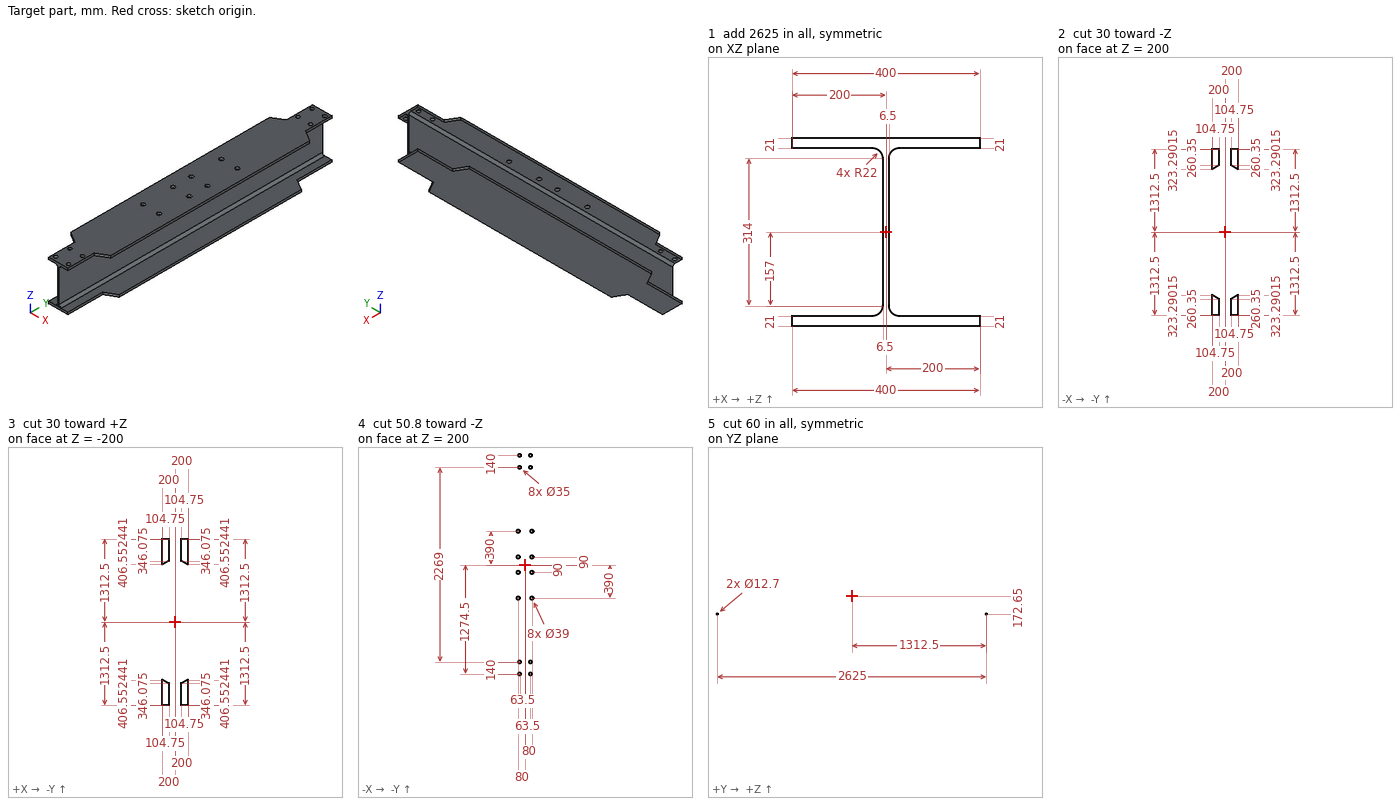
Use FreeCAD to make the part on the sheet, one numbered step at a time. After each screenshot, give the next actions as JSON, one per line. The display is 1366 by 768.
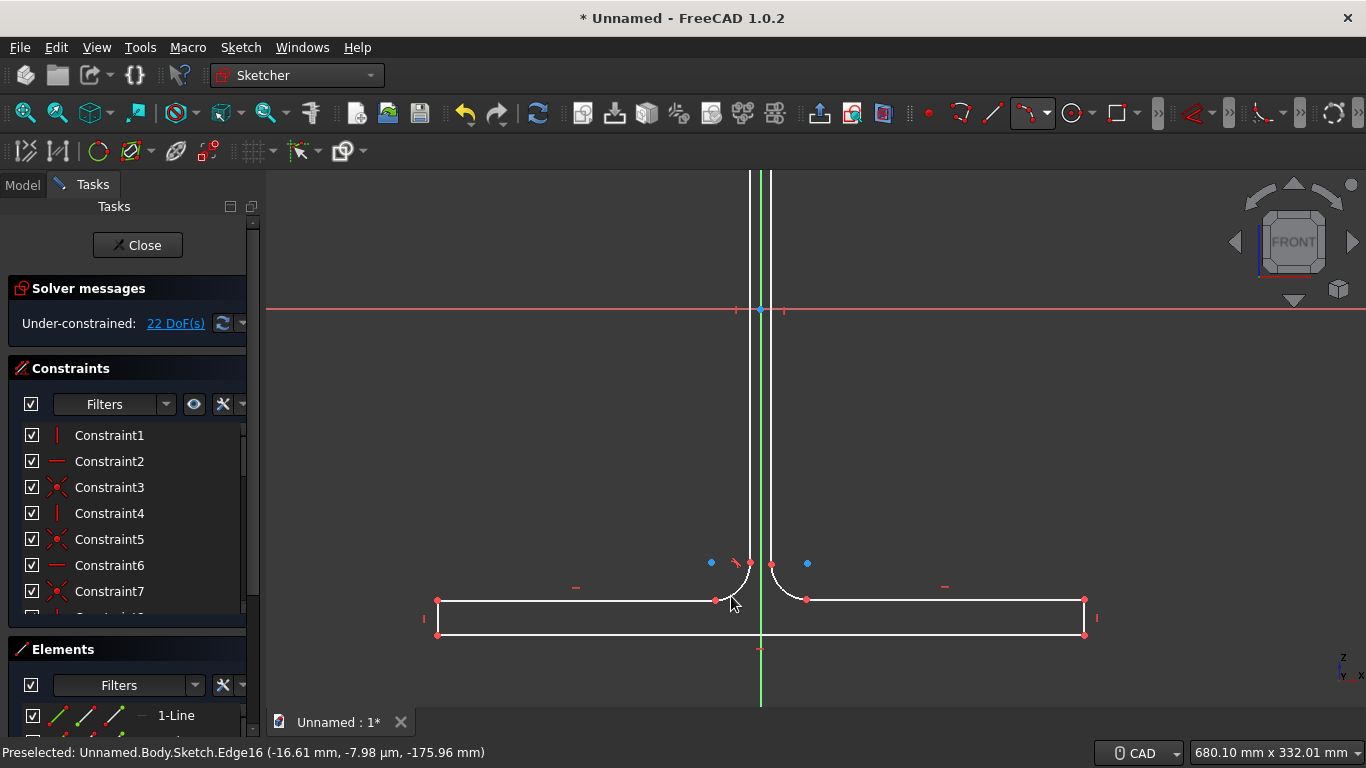
{"action": "scroll", "coordinate": [731, 596], "scroll_direction": "down", "scroll_amount": 3}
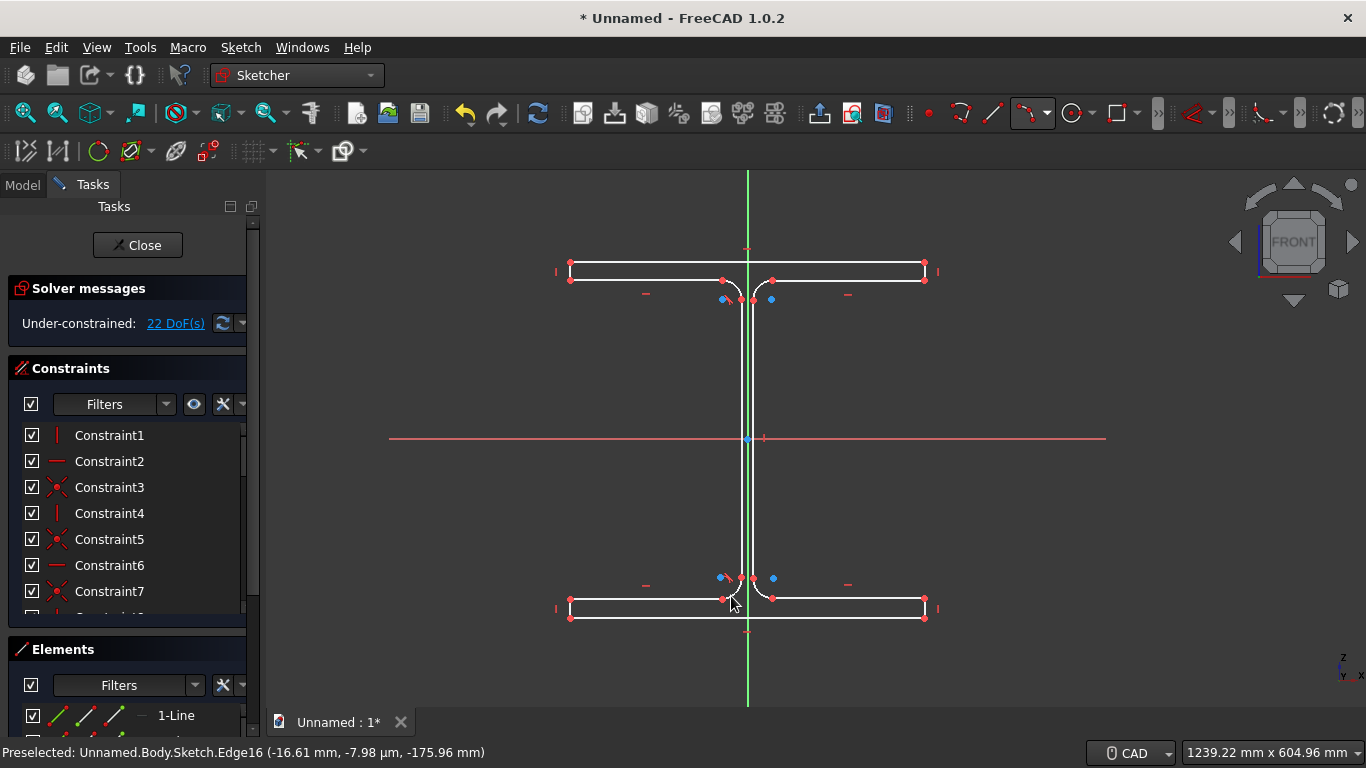
{"action": "left_click", "coordinate": [677, 280]}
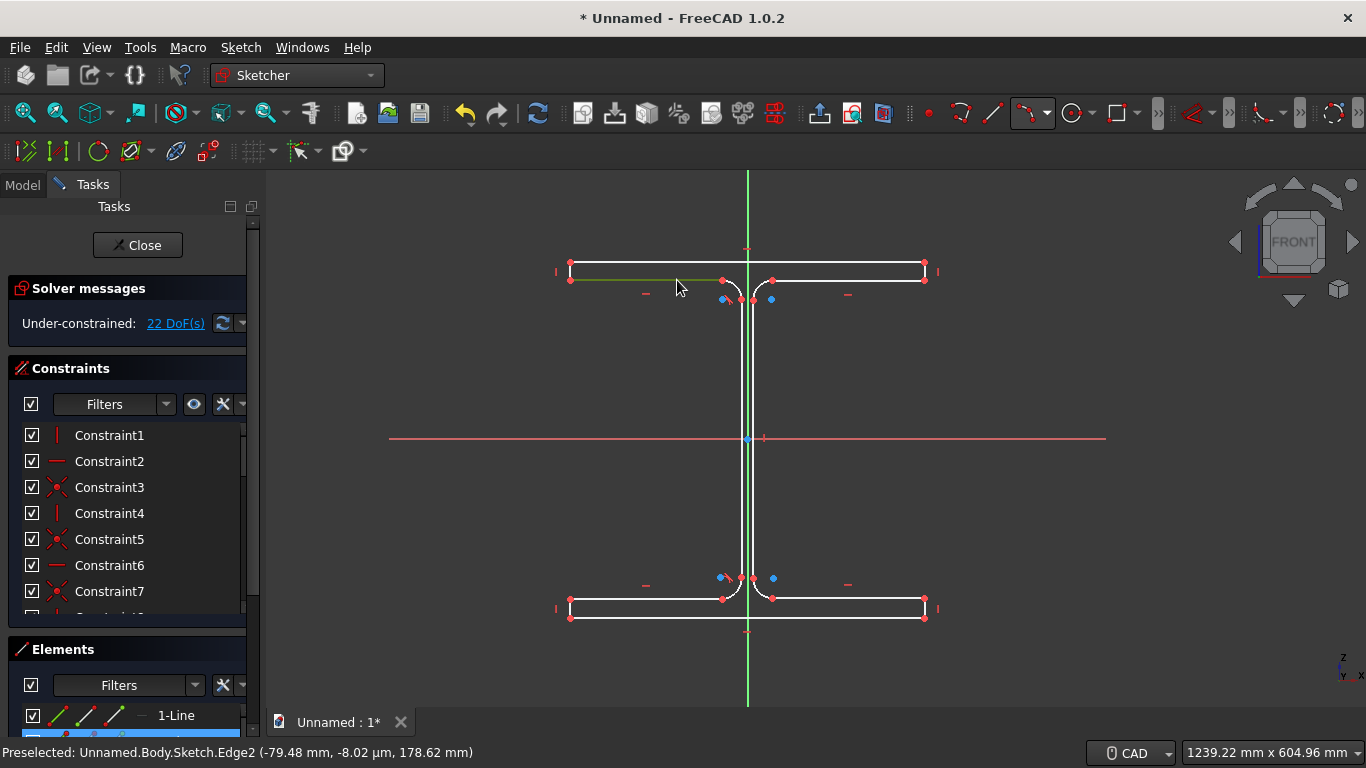
{"action": "scroll", "coordinate": [731, 283], "scroll_direction": "up", "scroll_amount": 3}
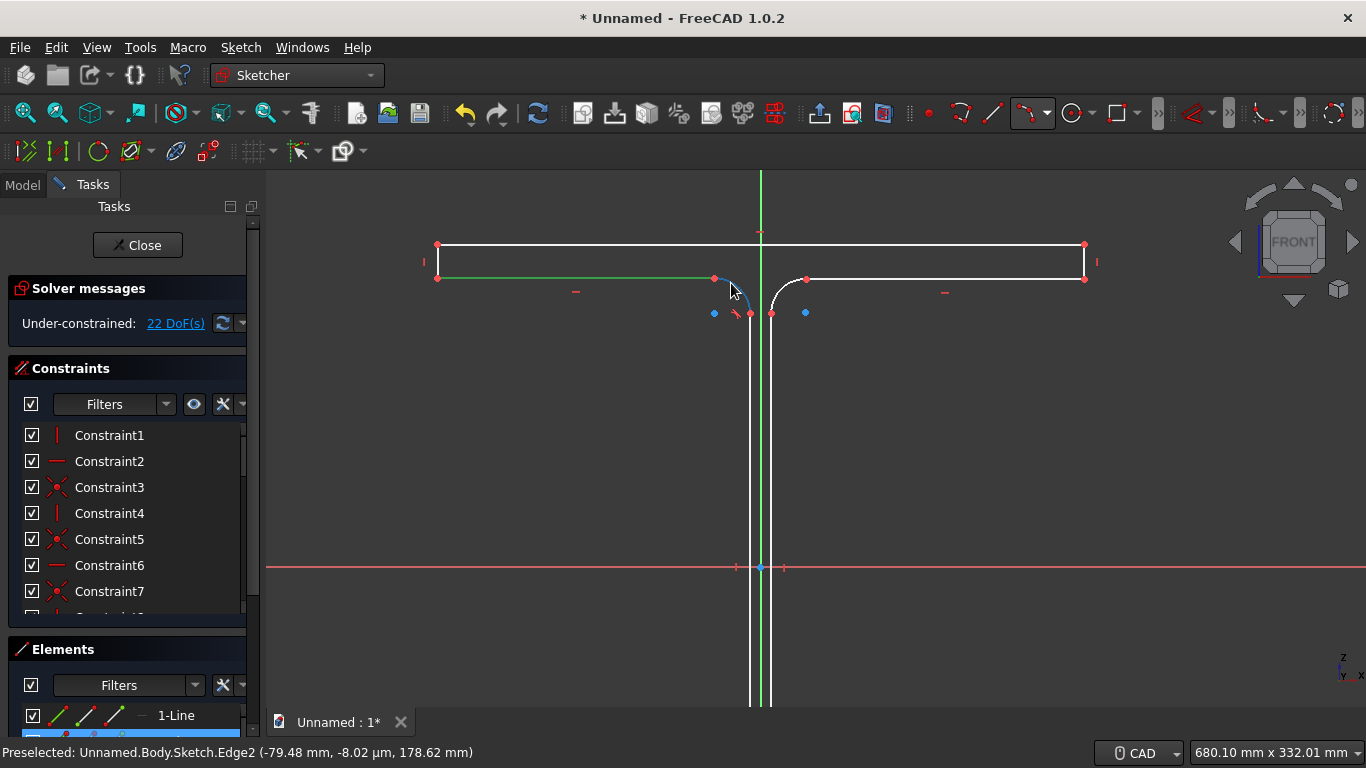
{"action": "left_click", "coordinate": [731, 282]}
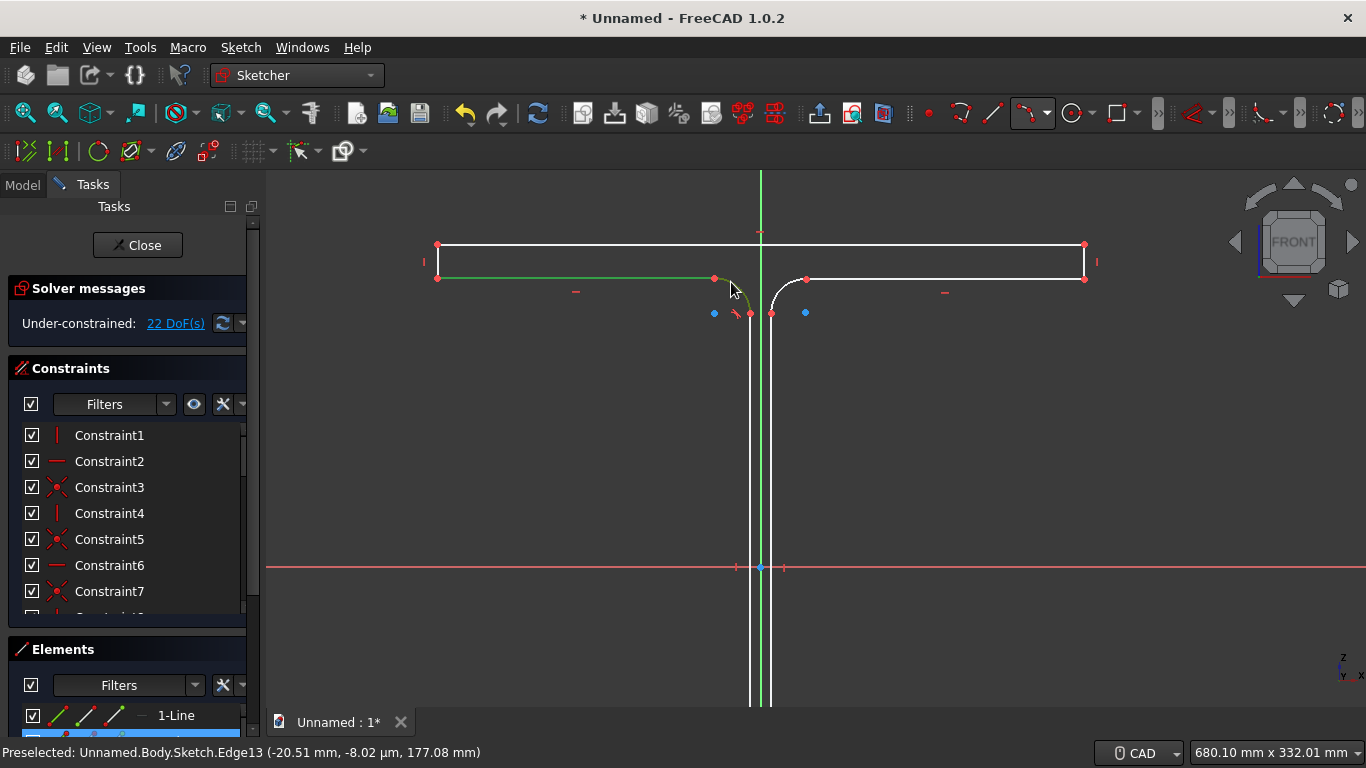
{"action": "key", "text": "t"}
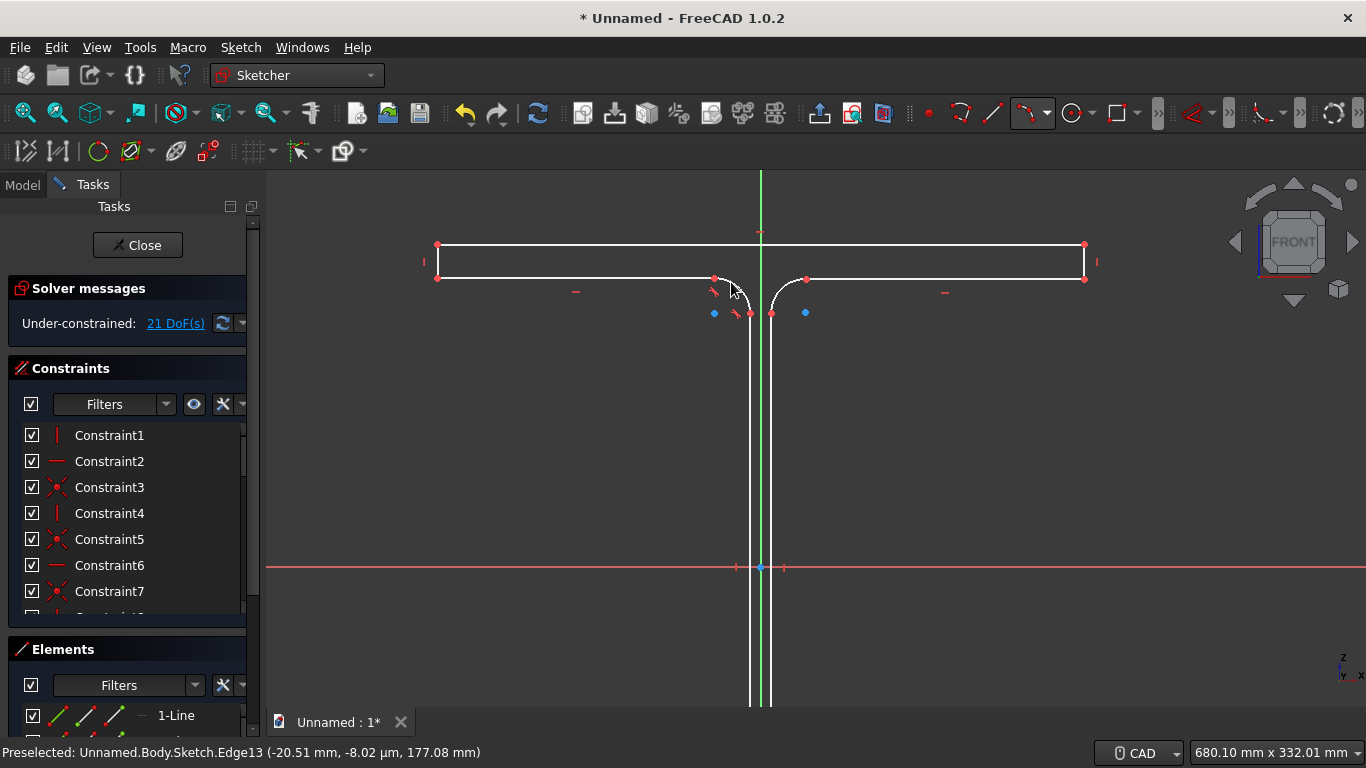
{"action": "left_click", "coordinate": [1001, 279]}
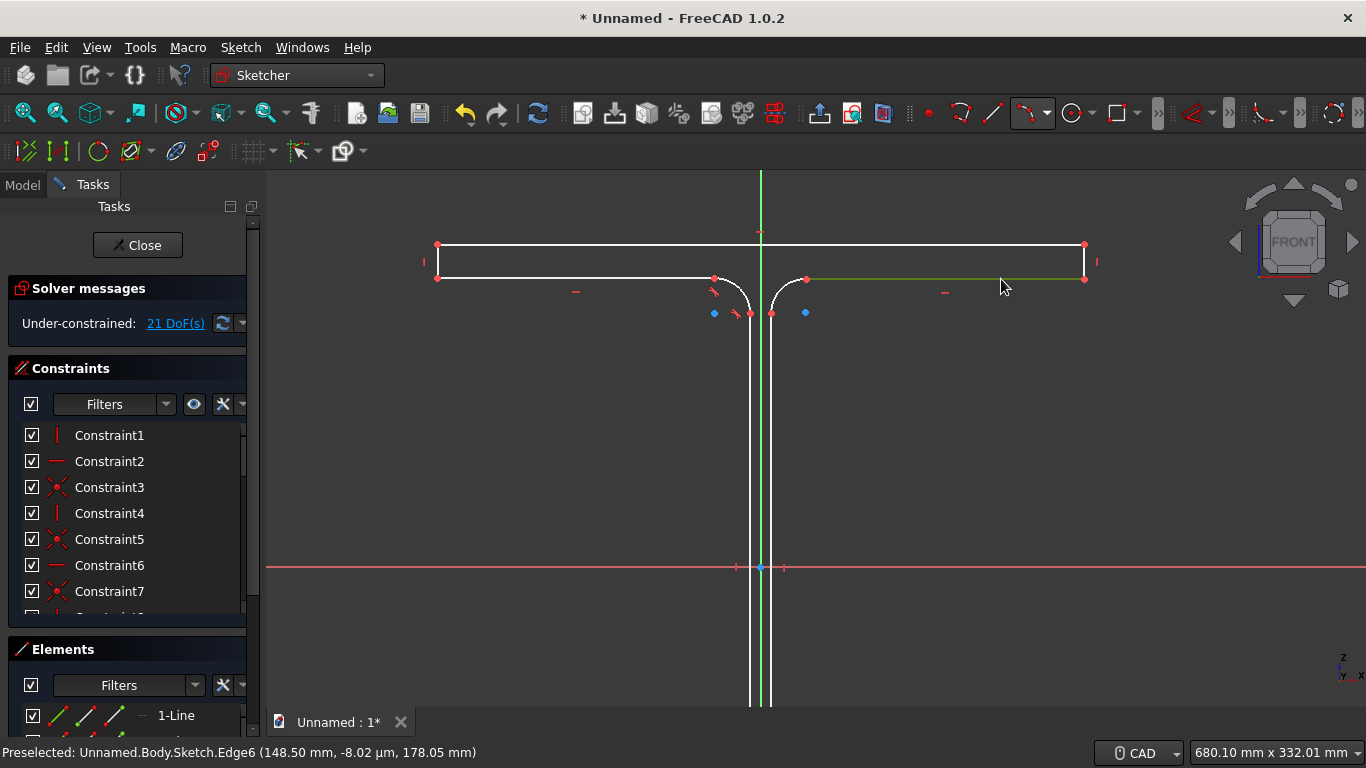
{"action": "left_click", "coordinate": [790, 283]}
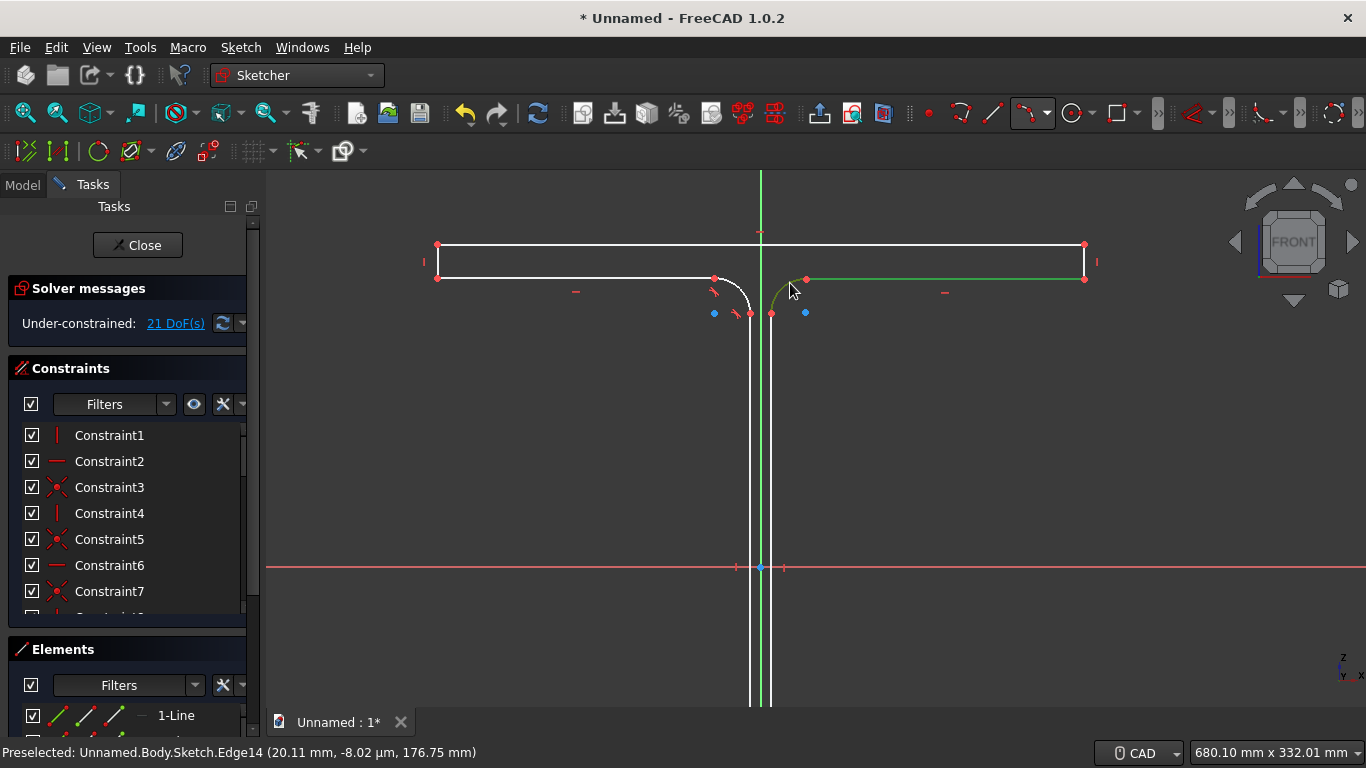
{"action": "key", "text": "t"}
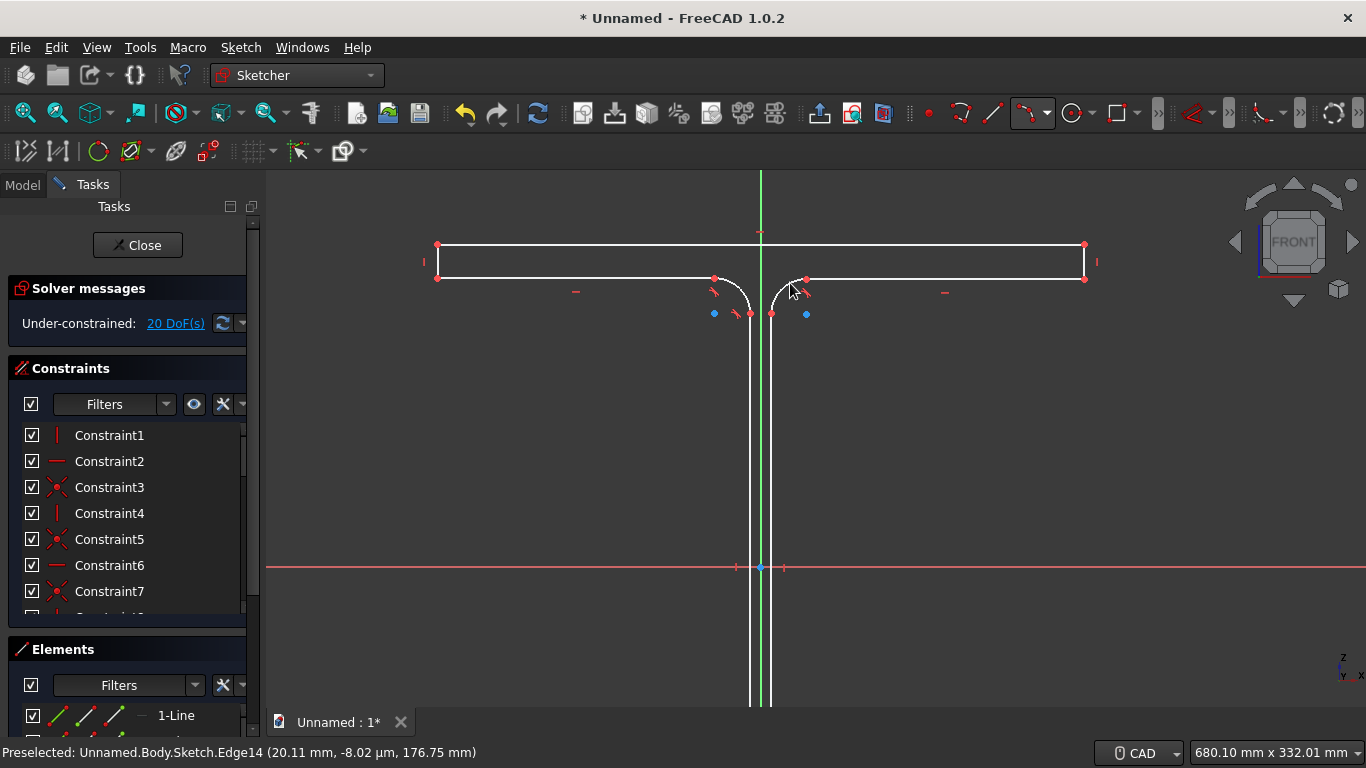
{"action": "scroll", "coordinate": [771, 466], "scroll_direction": "up", "scroll_amount": 2}